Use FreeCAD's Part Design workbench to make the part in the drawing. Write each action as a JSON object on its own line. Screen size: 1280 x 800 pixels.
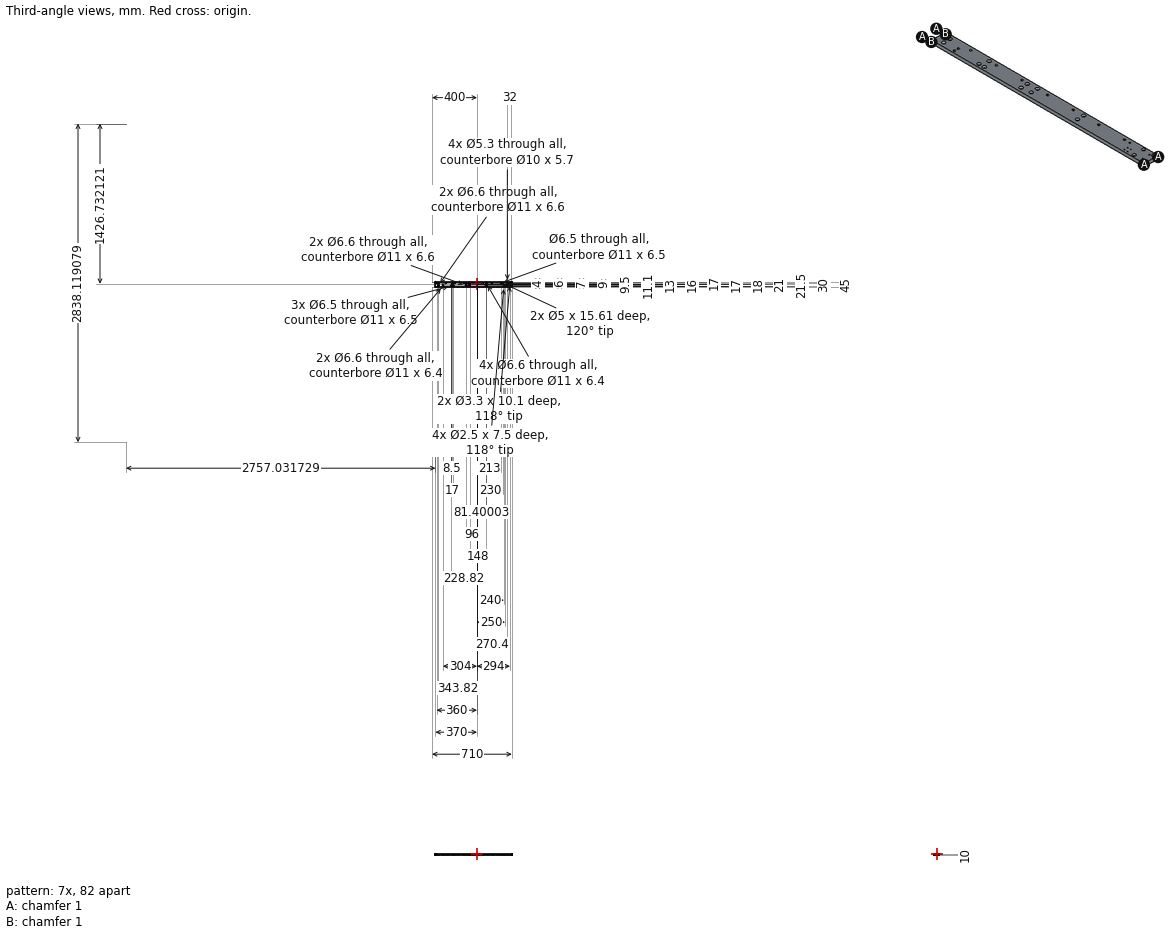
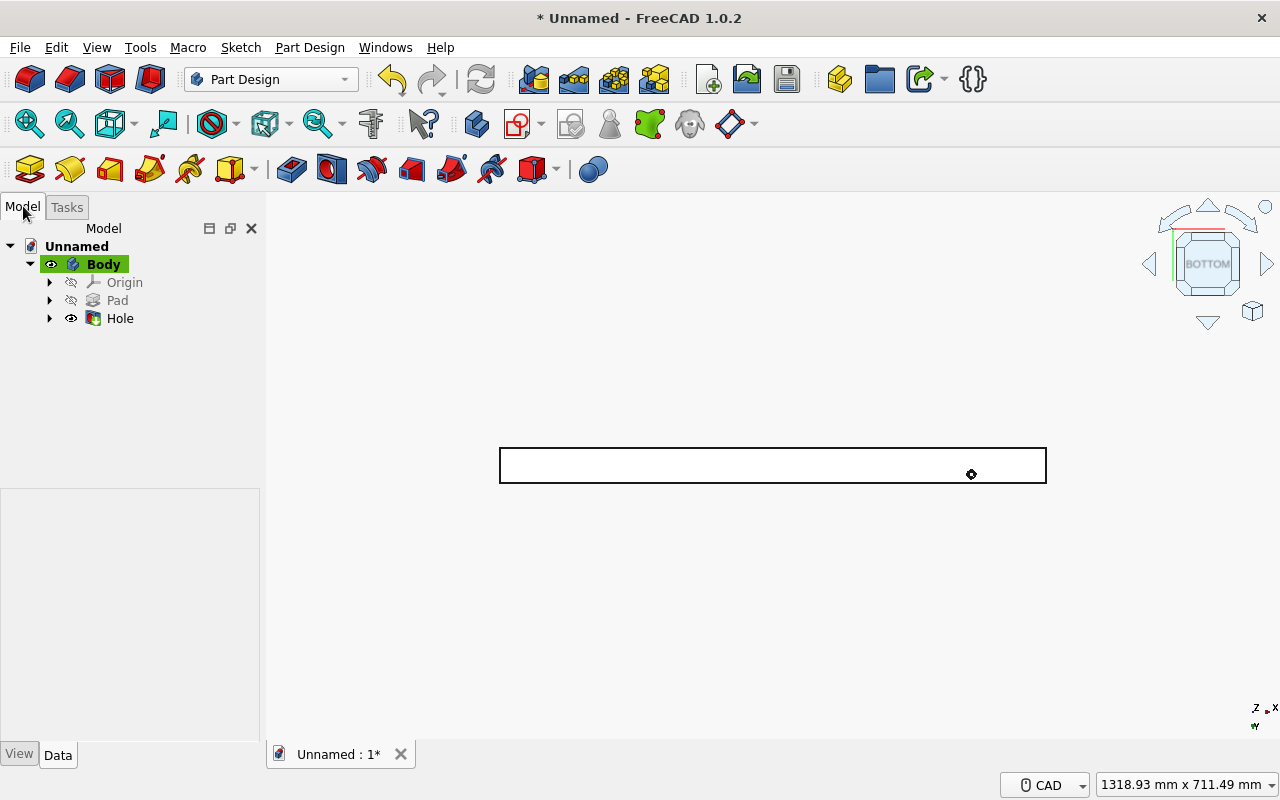
{"action": "left_click", "coordinate": [116, 318]}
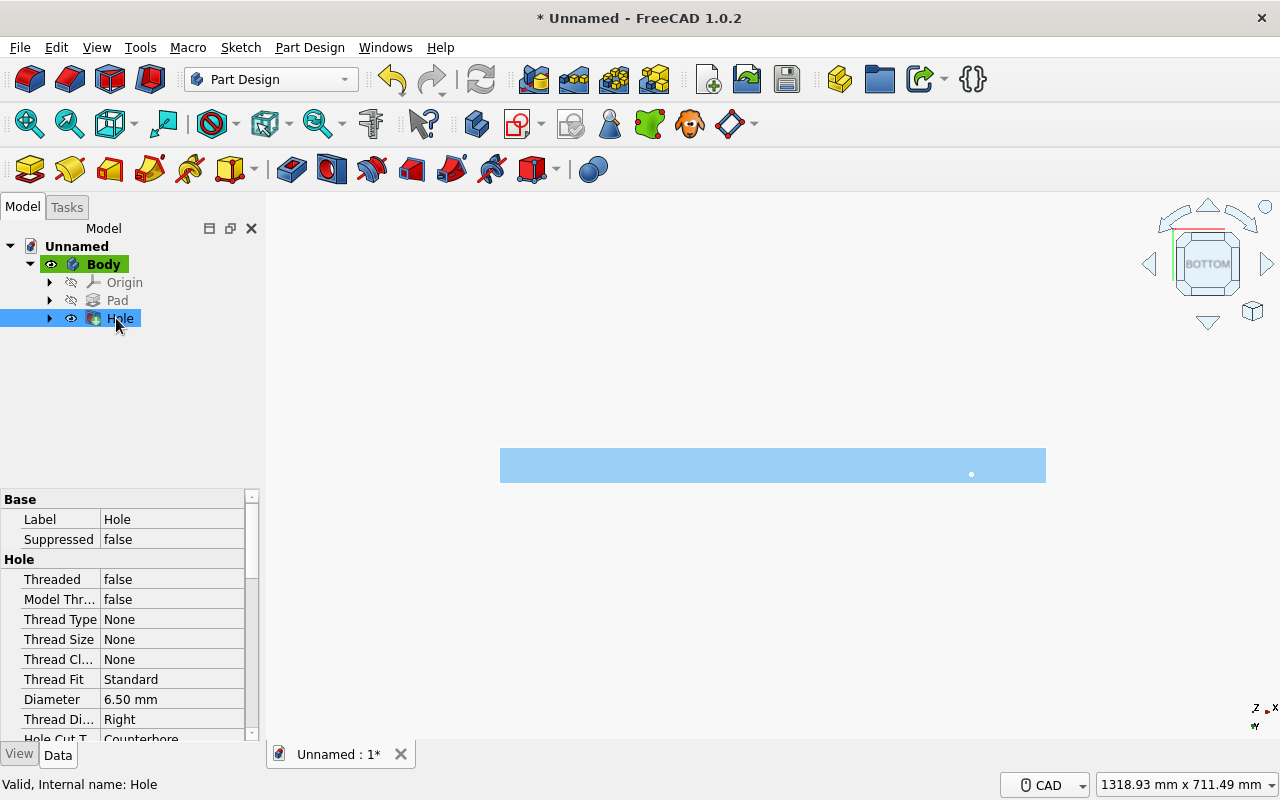
{"action": "left_click", "coordinate": [574, 80]}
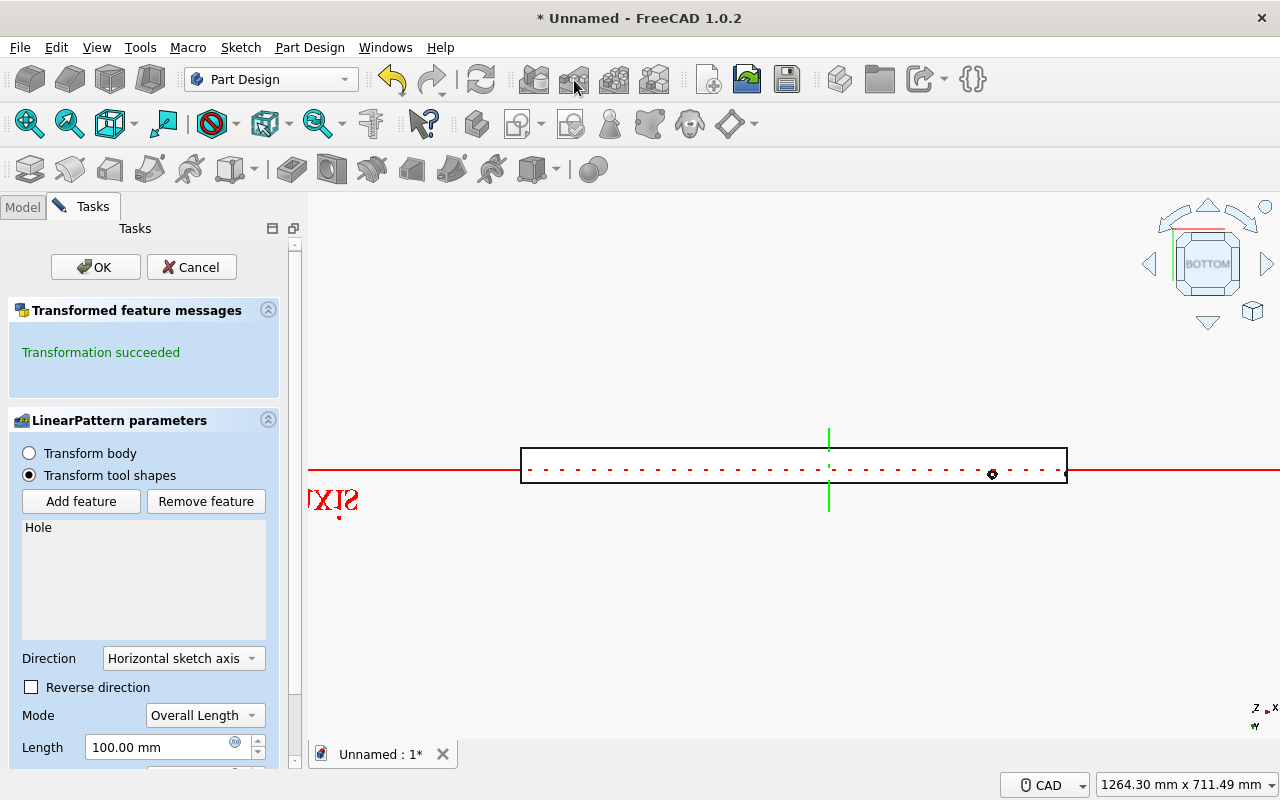
{"action": "left_click", "coordinate": [184, 658]}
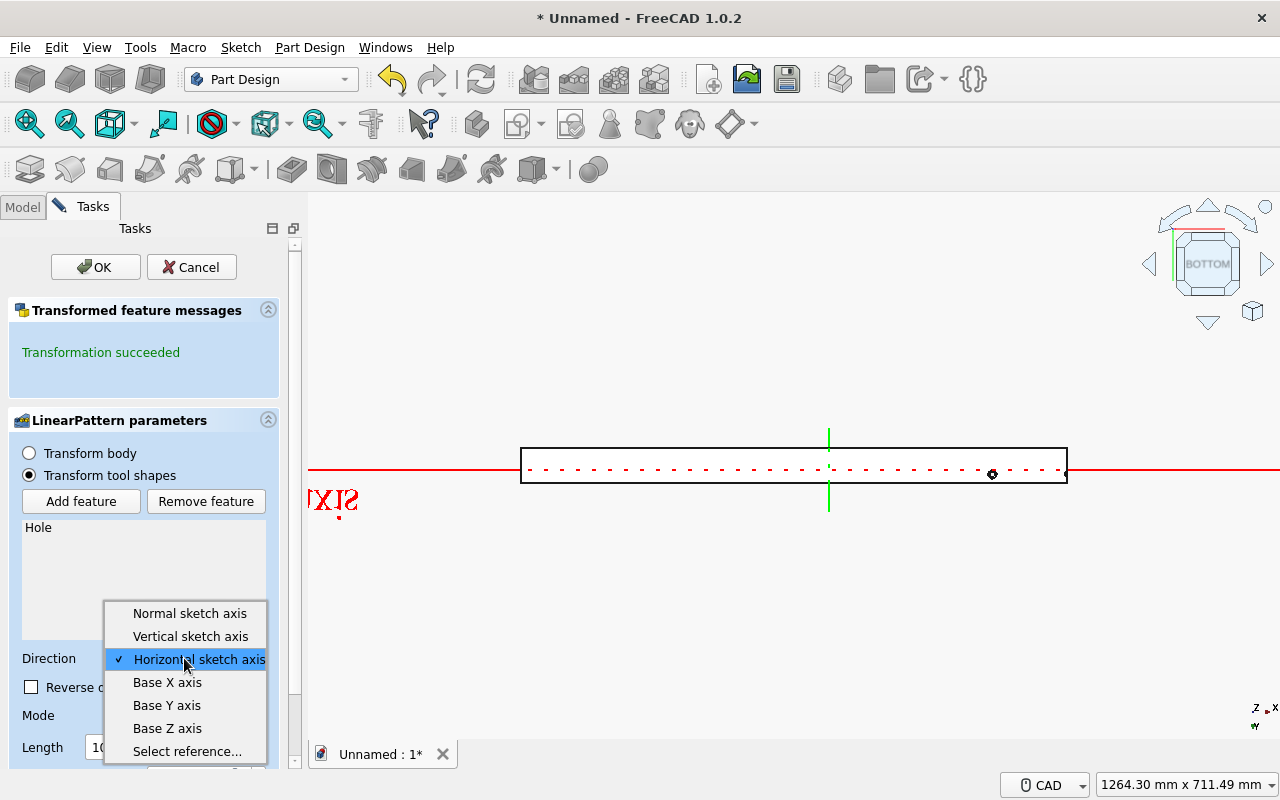
{"action": "left_click", "coordinate": [184, 682]}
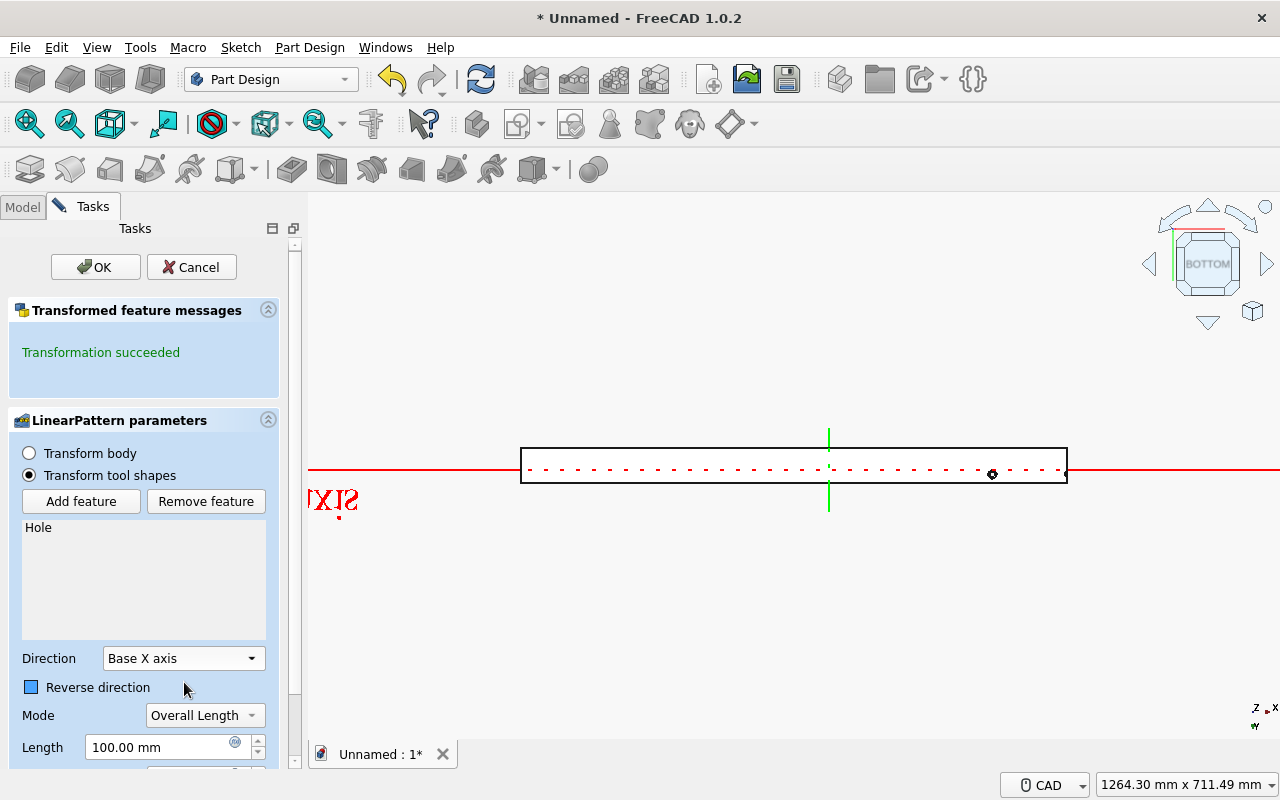
{"action": "left_click", "coordinate": [206, 716]}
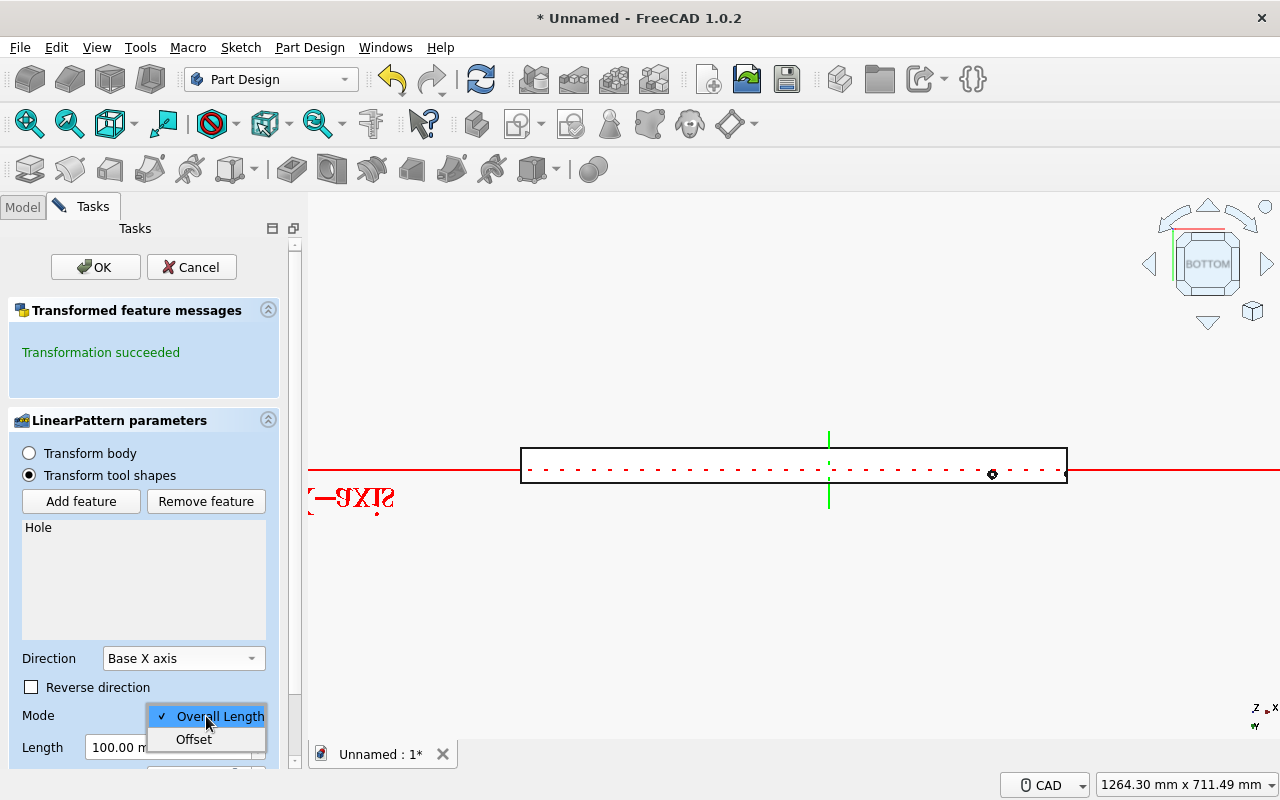
{"action": "left_click", "coordinate": [206, 740]}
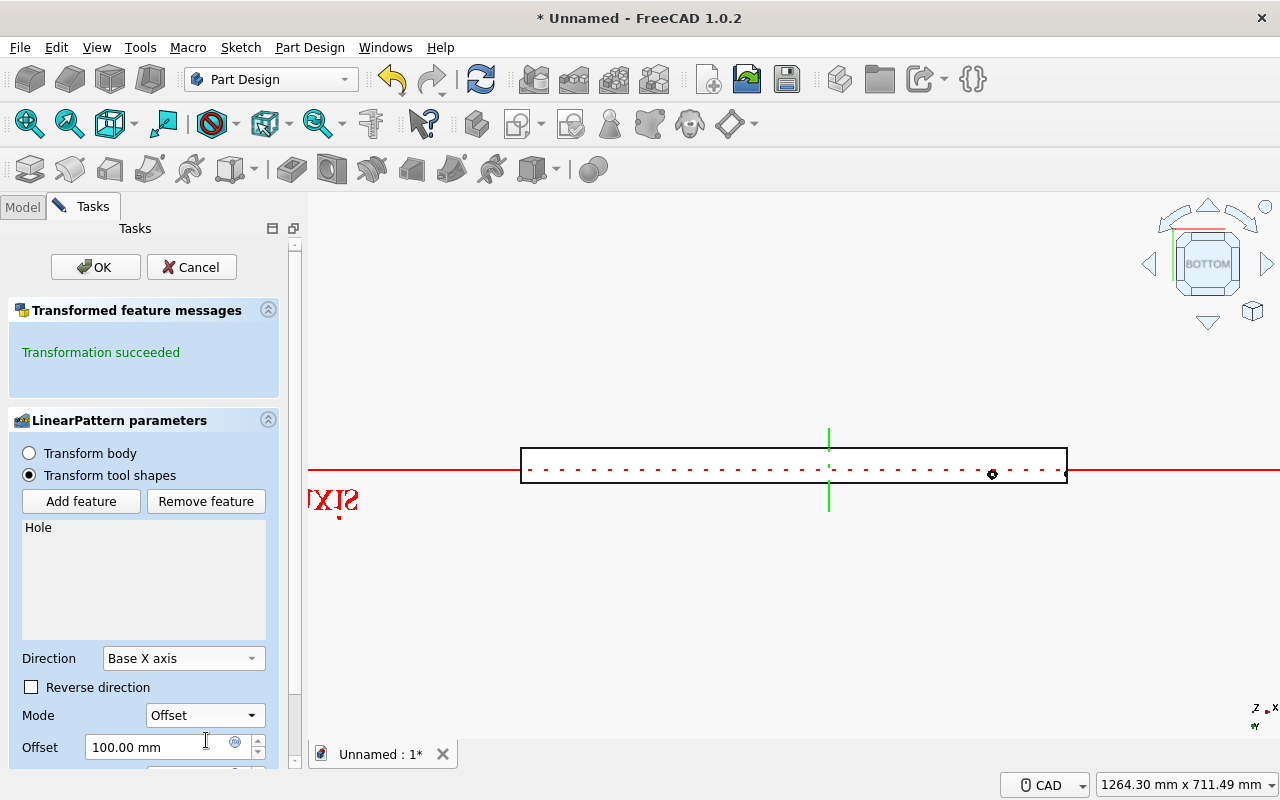
{"action": "triple_click", "coordinate": [168, 747]}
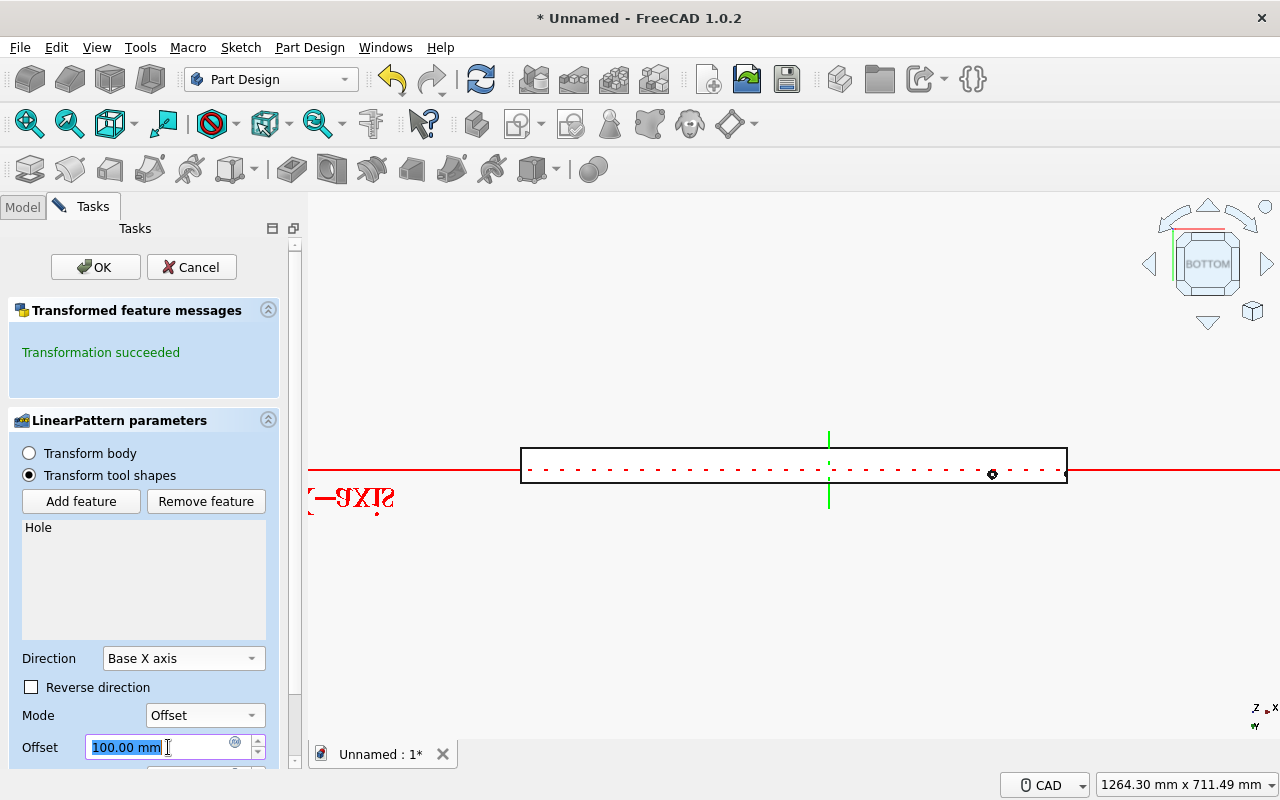
{"action": "type", "text": "82"}
{"action": "key", "text": "Tab"}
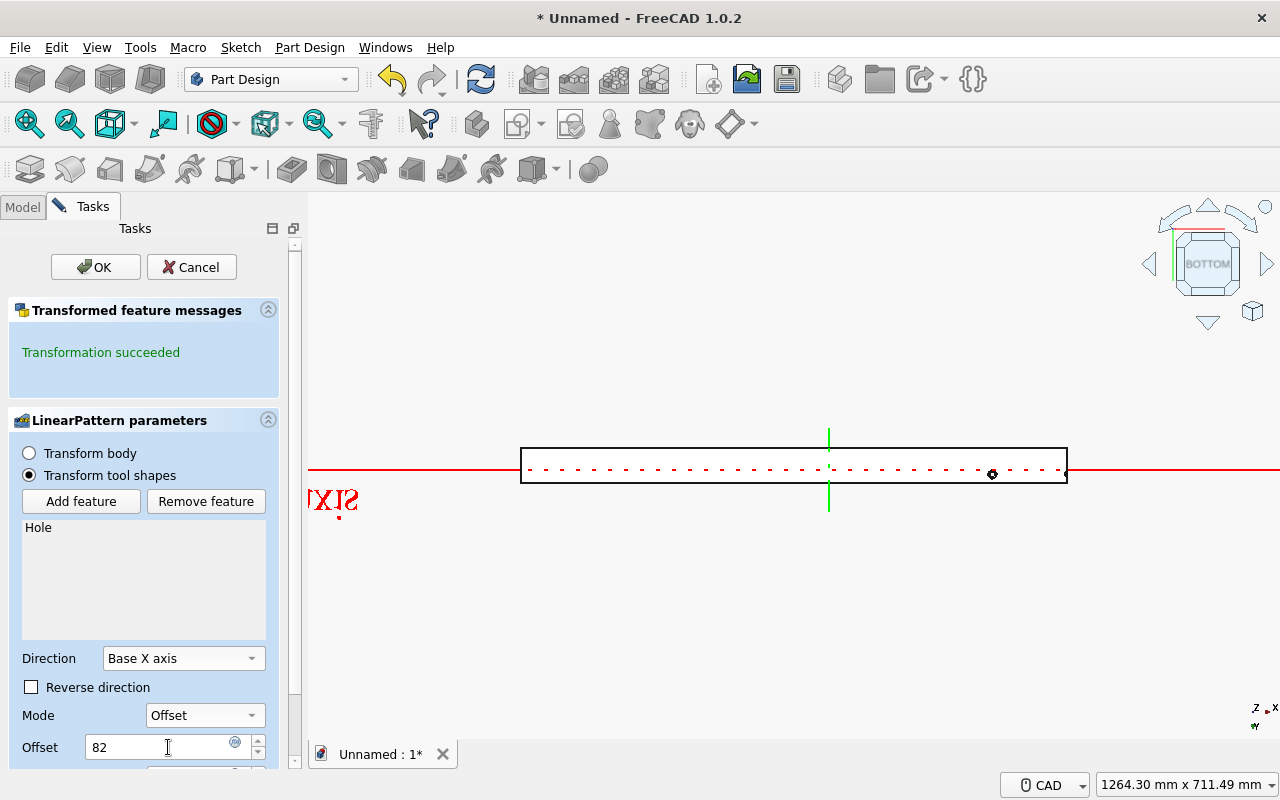
{"action": "scroll", "coordinate": [295, 503], "scroll_direction": "down", "scroll_amount": 2}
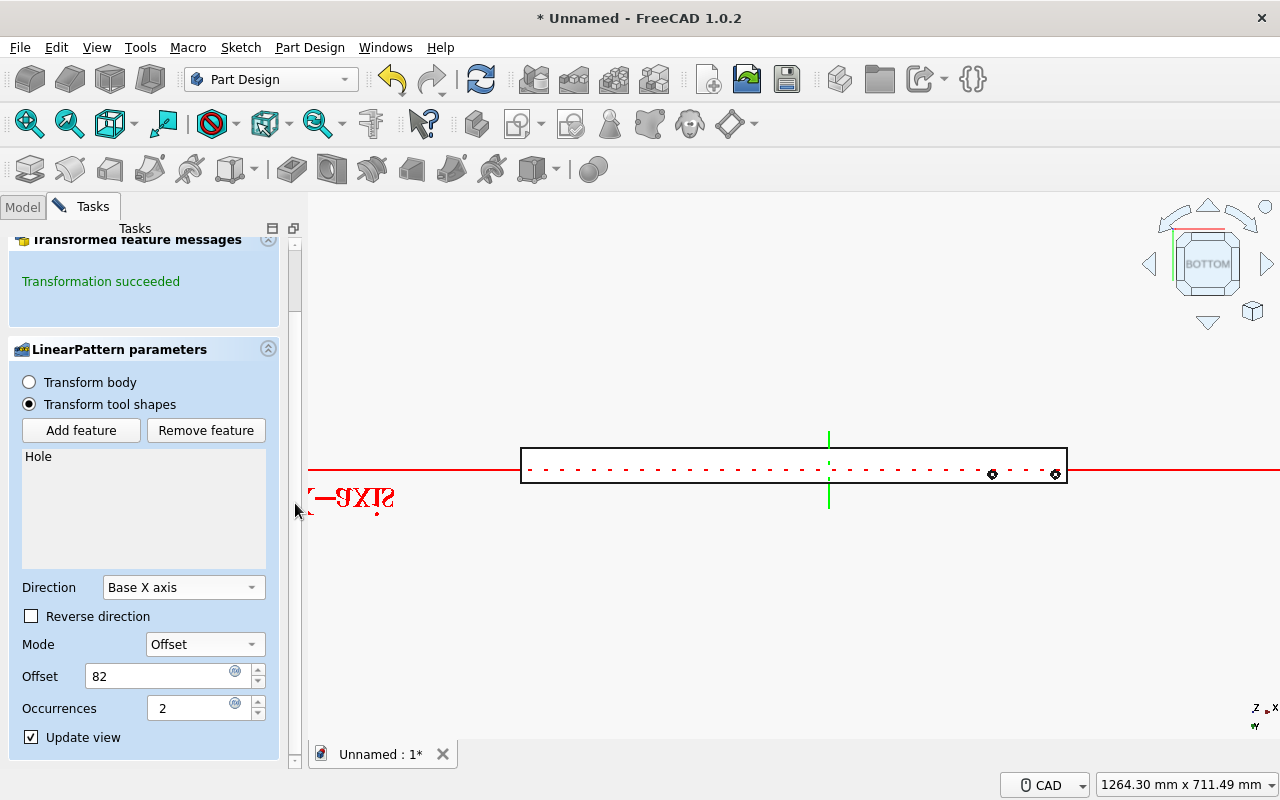
{"action": "triple_click", "coordinate": [198, 708]}